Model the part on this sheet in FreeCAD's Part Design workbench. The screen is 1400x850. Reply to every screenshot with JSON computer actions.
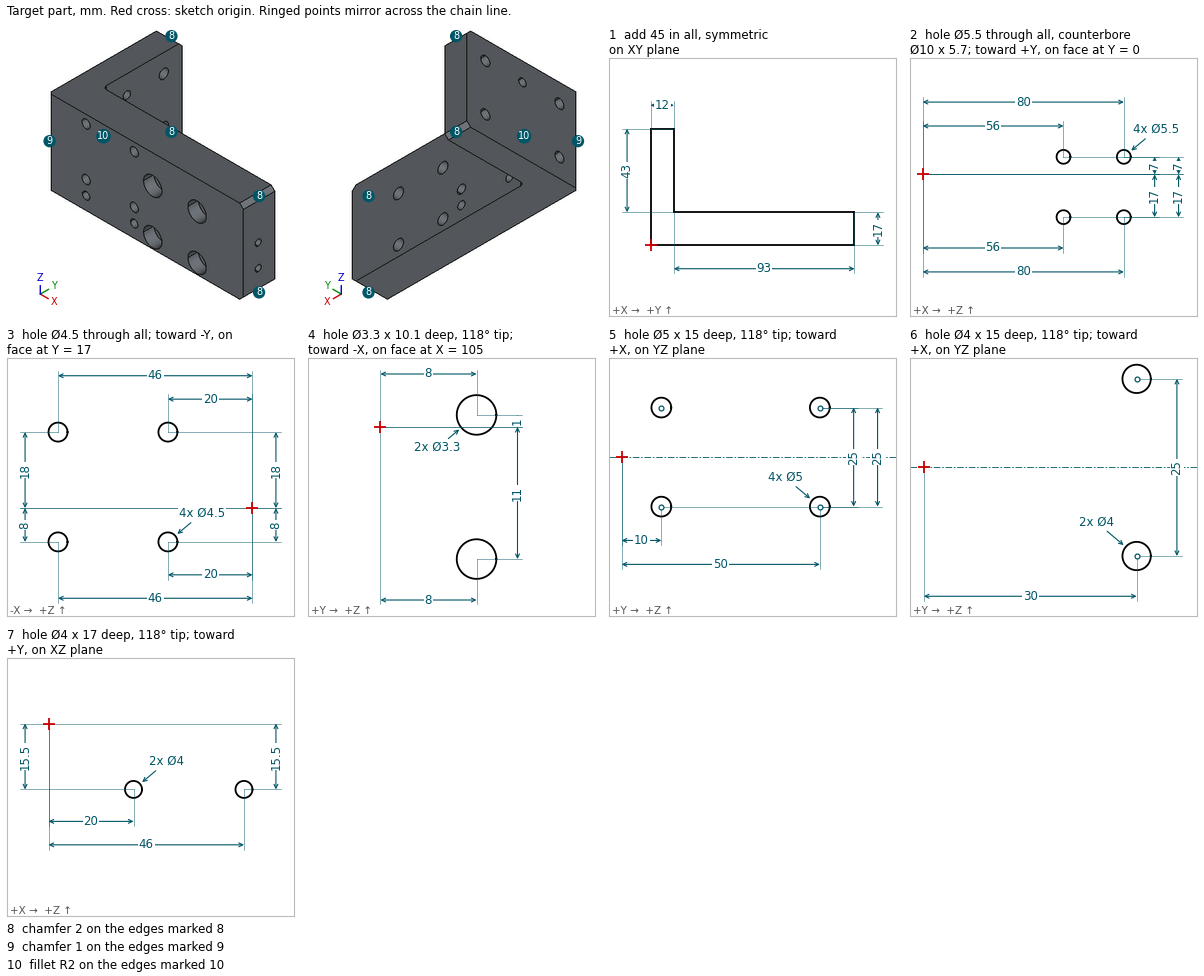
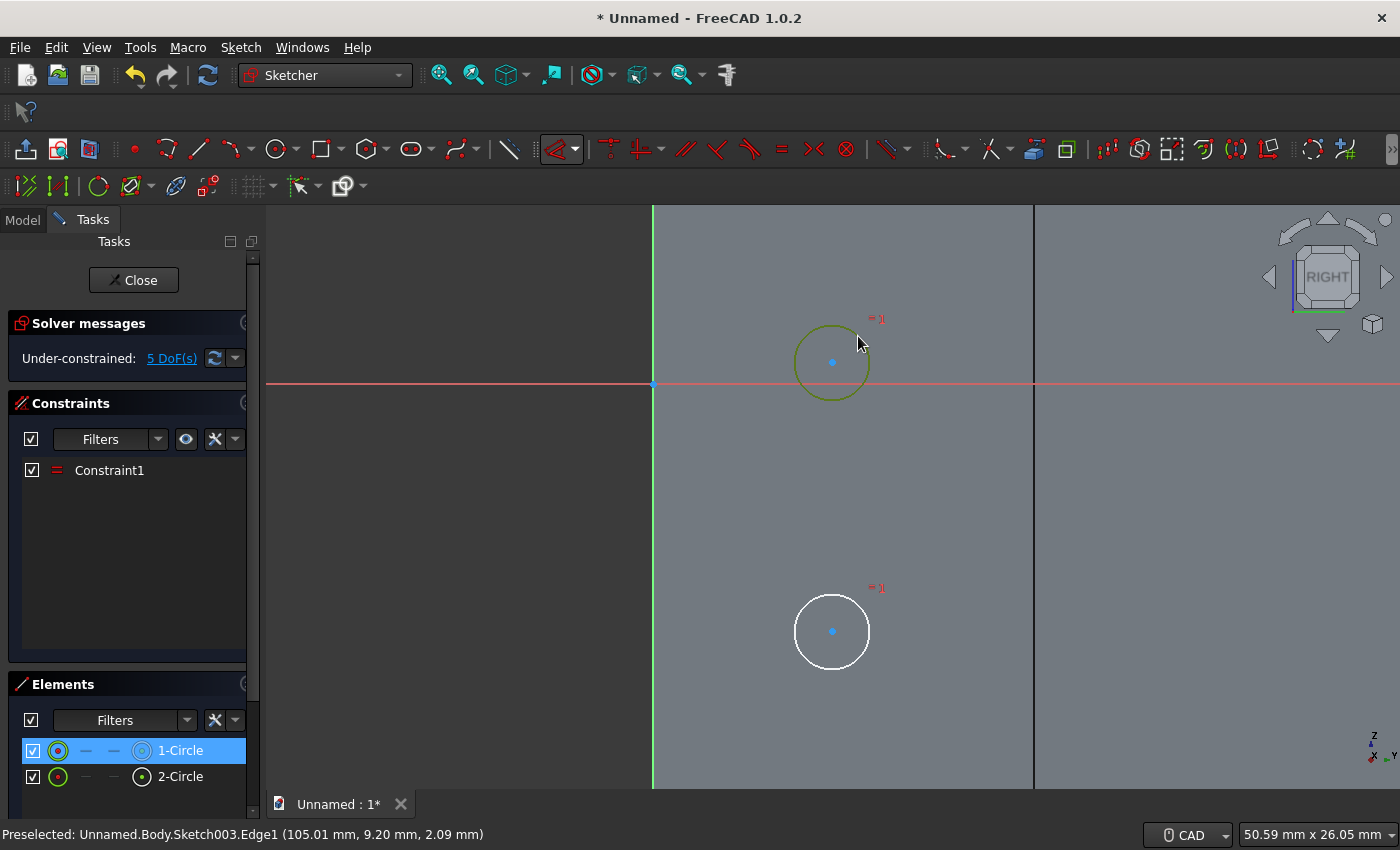
{"action": "left_click", "coordinate": [578, 150]}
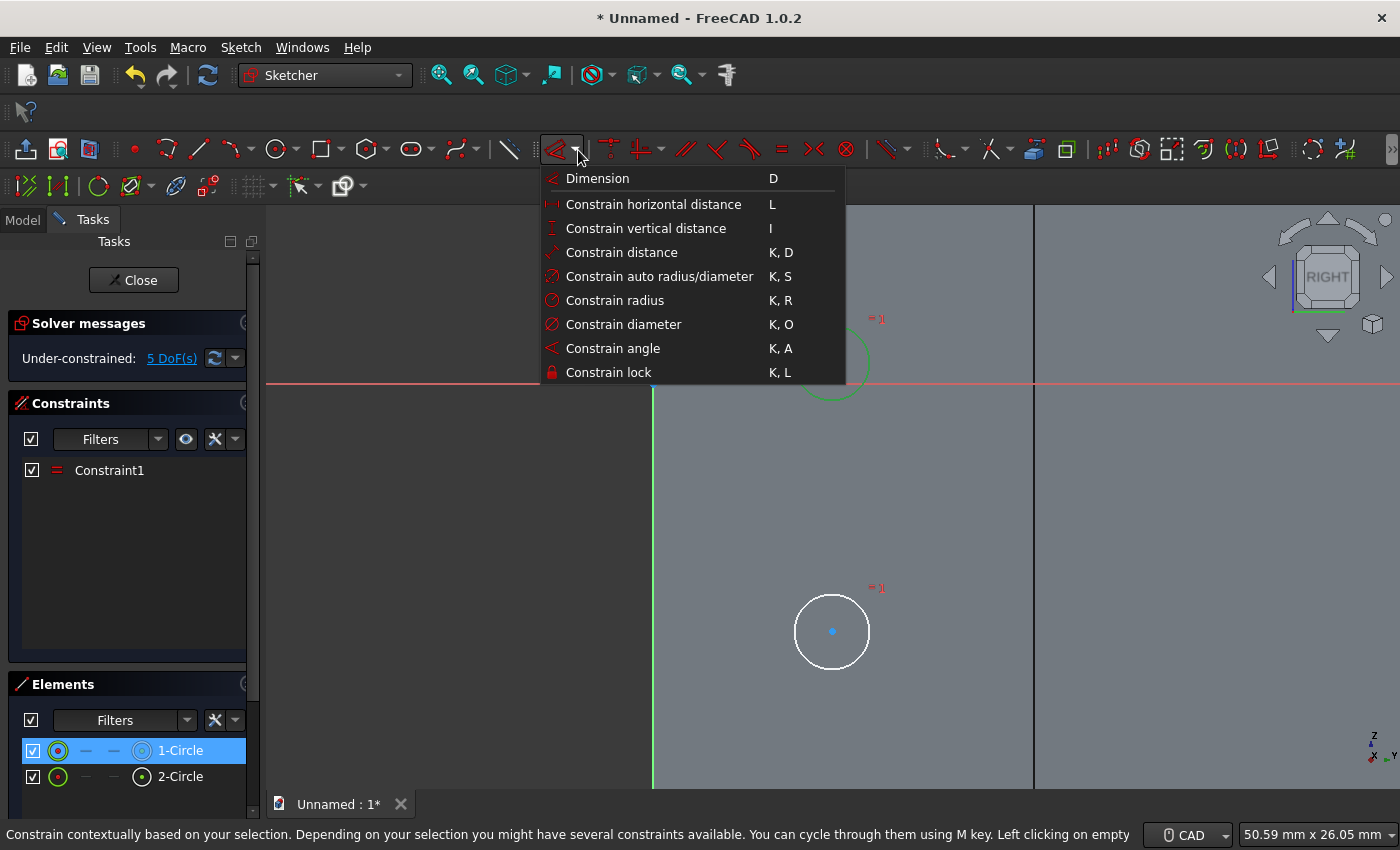
{"action": "left_click", "coordinate": [693, 324]}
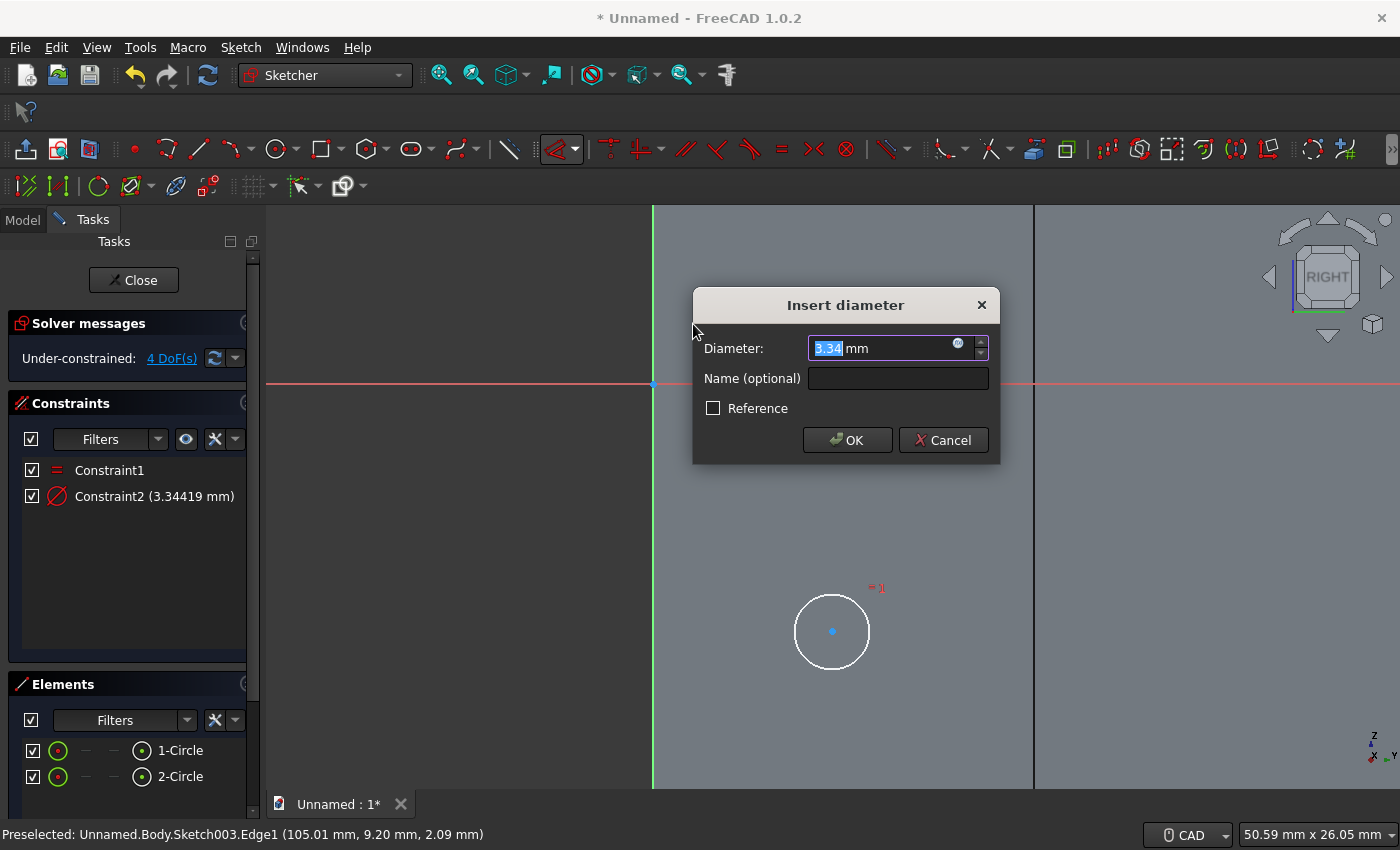
{"action": "type", "text": "3.3"}
{"action": "key", "text": "Return"}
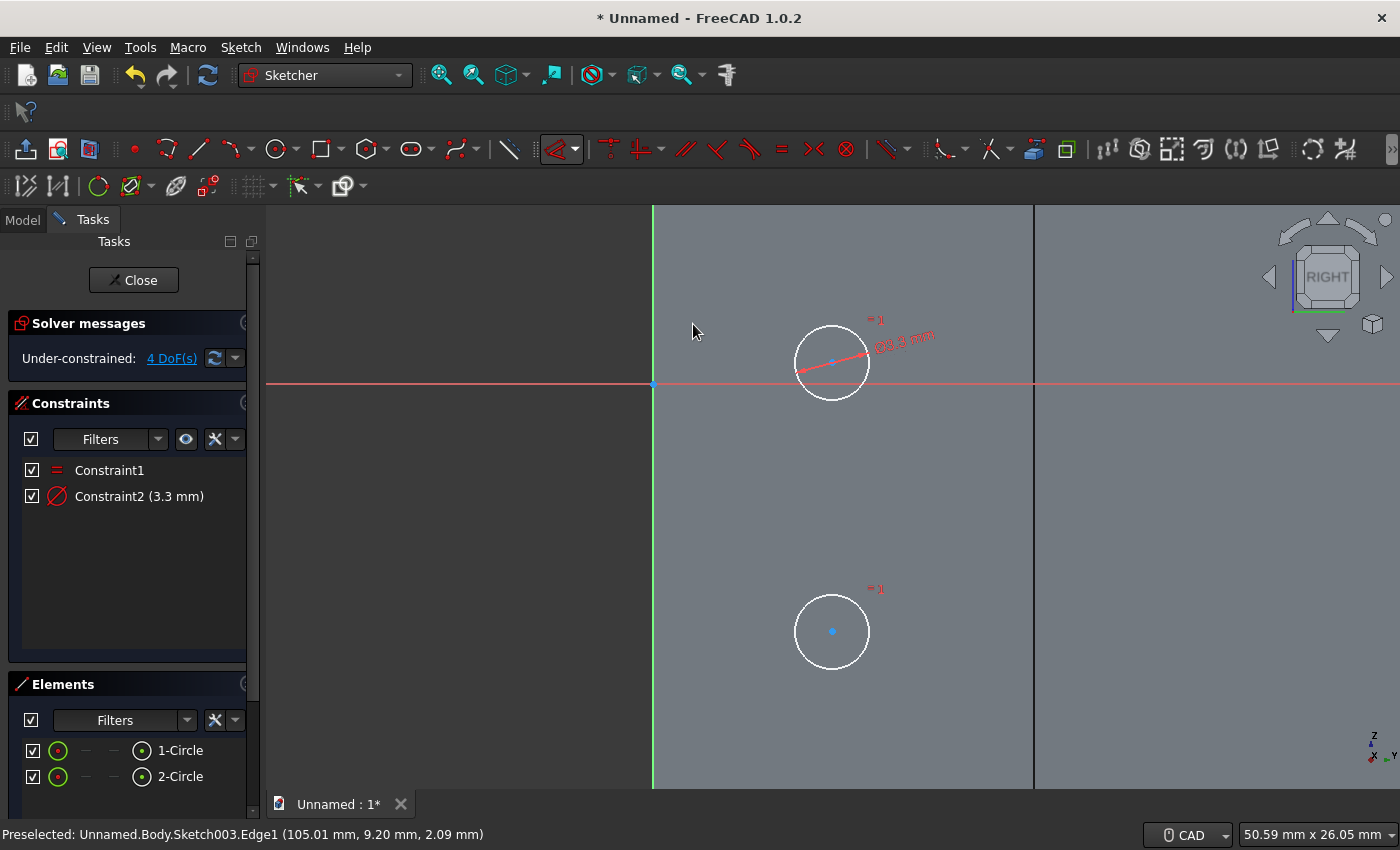
{"action": "left_click", "coordinate": [832, 363]}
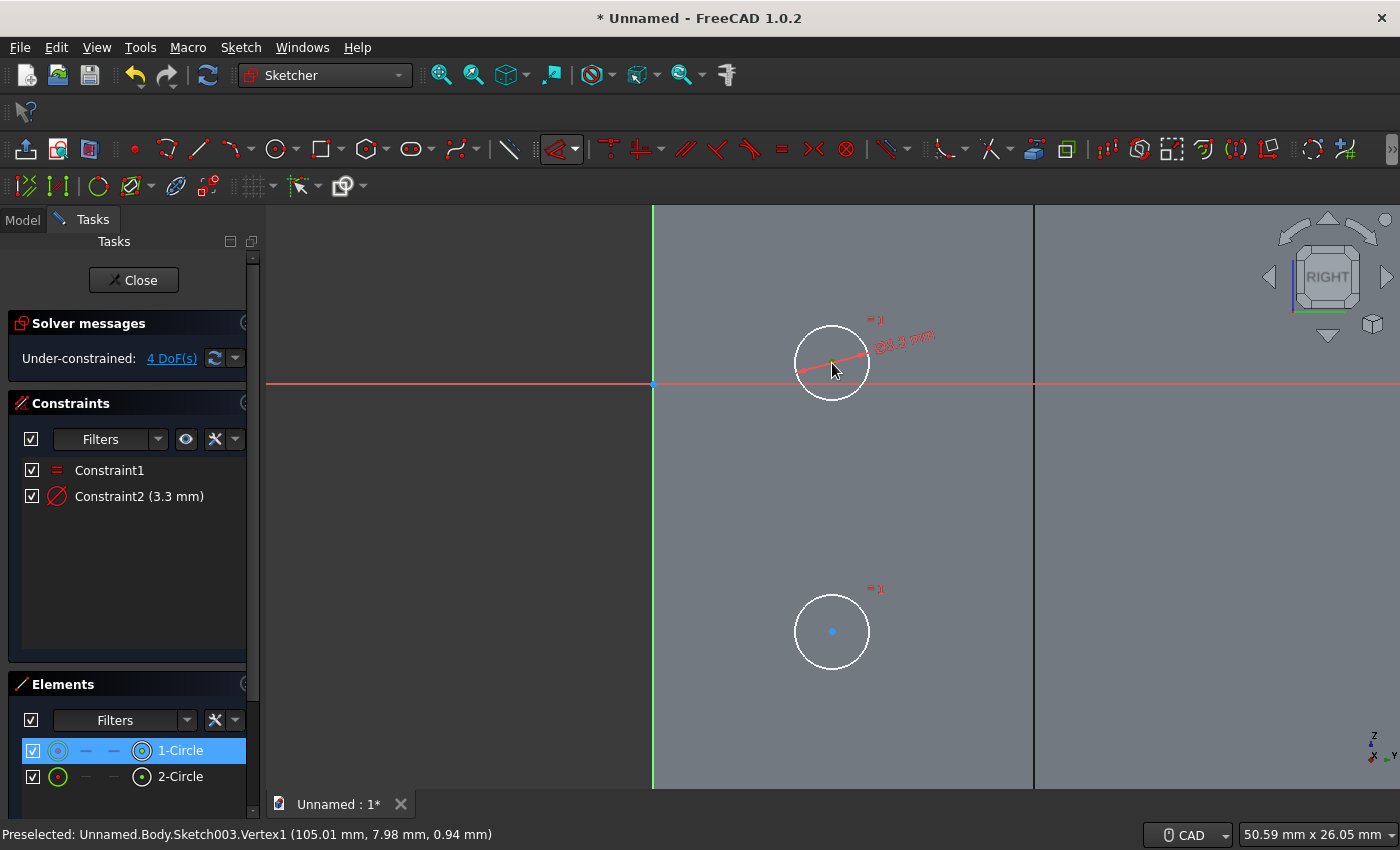
{"action": "left_click", "coordinate": [578, 150]}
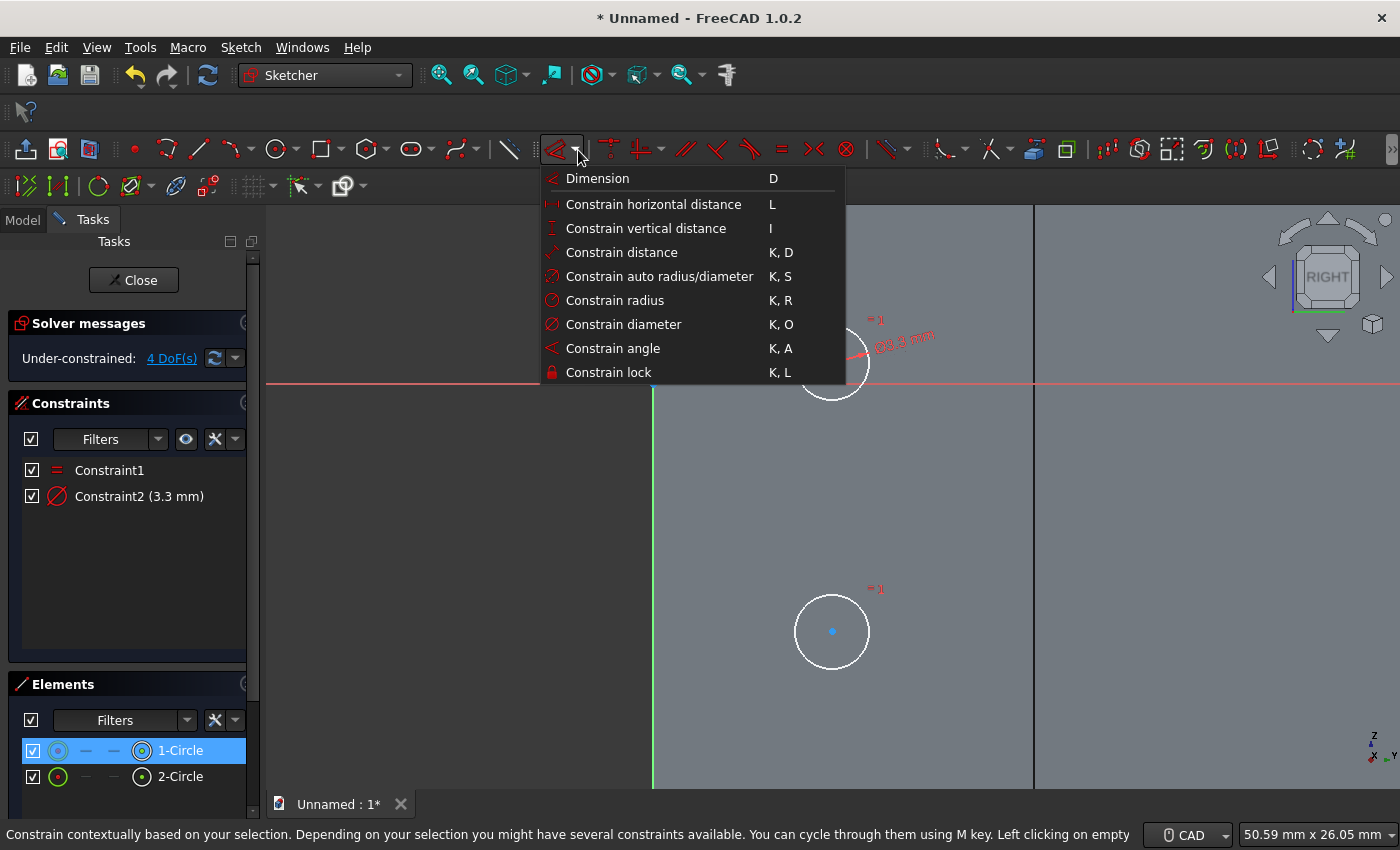
{"action": "left_click", "coordinate": [693, 204]}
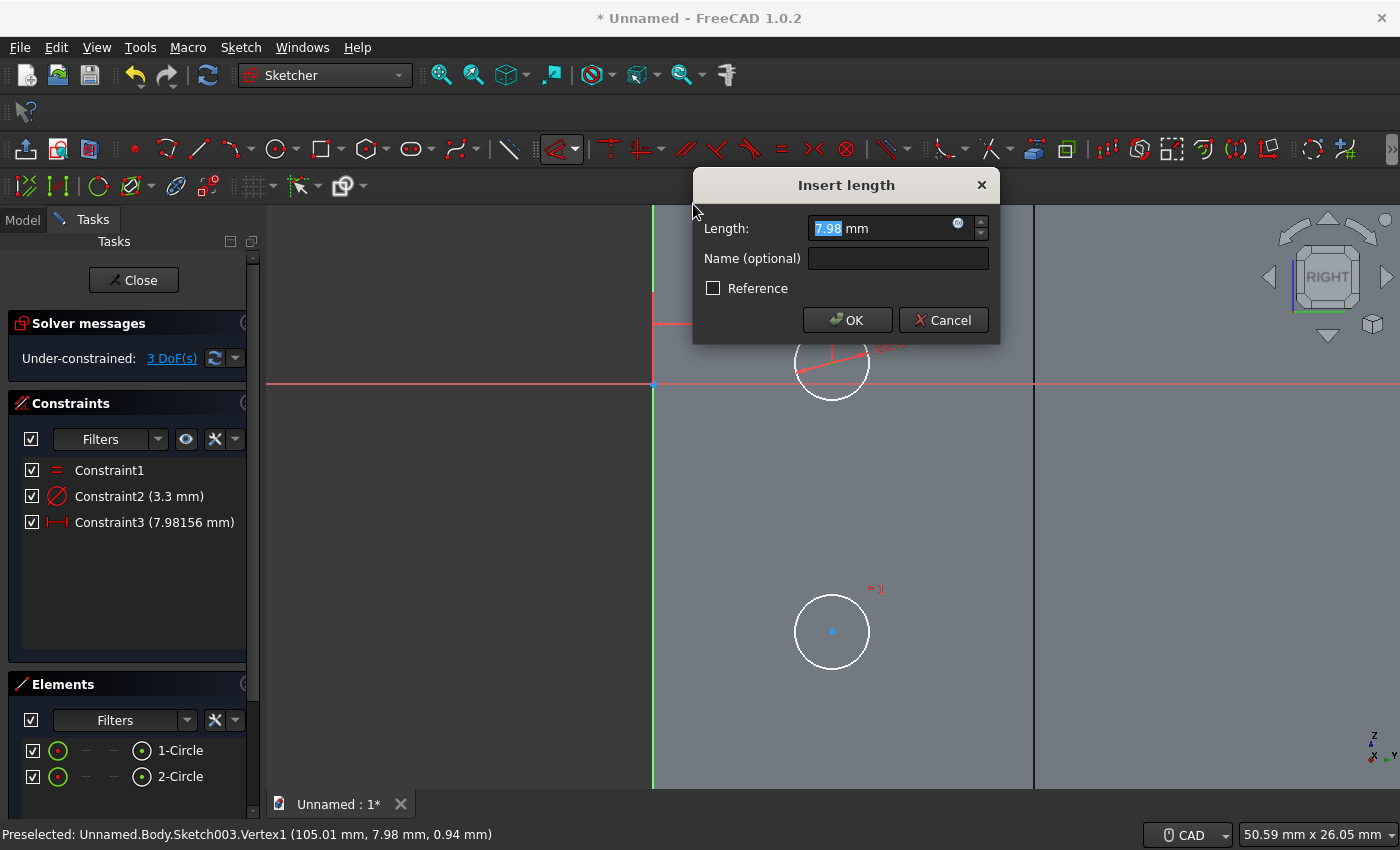
{"action": "type", "text": "8"}
{"action": "key", "text": "Return"}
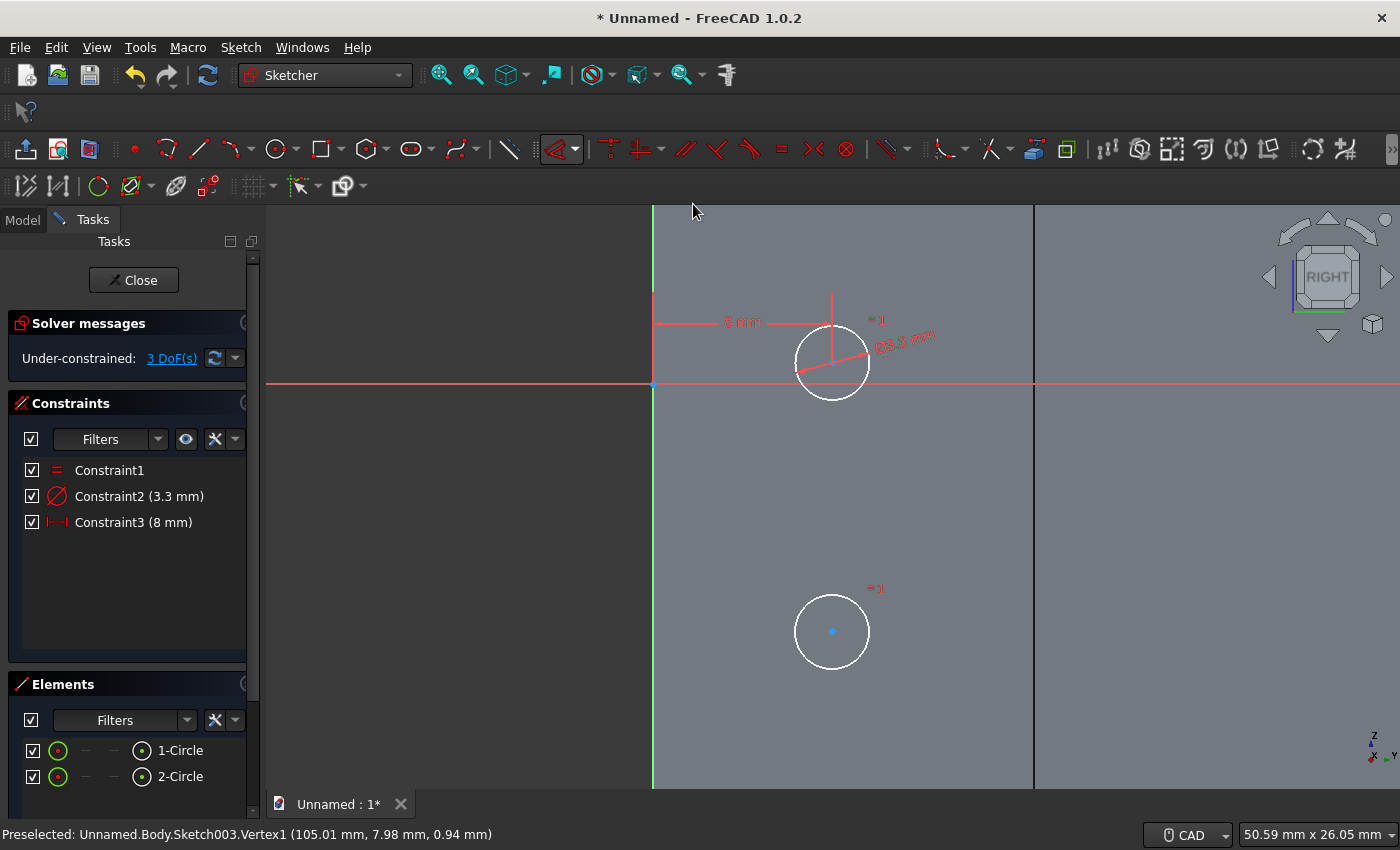
{"action": "scroll", "coordinate": [832, 363], "scroll_direction": "up", "scroll_amount": 3}